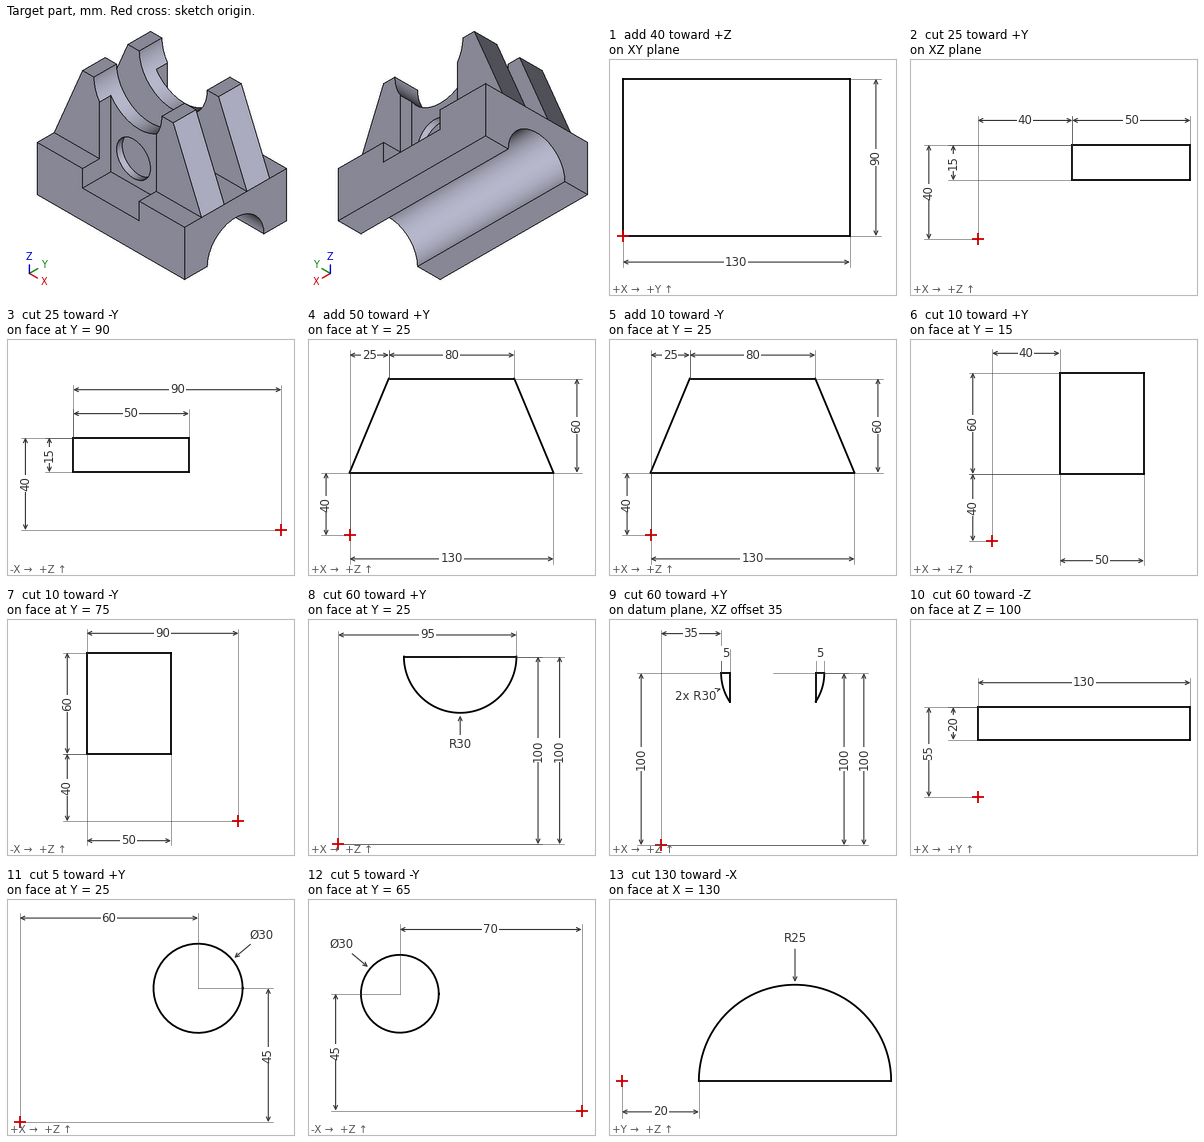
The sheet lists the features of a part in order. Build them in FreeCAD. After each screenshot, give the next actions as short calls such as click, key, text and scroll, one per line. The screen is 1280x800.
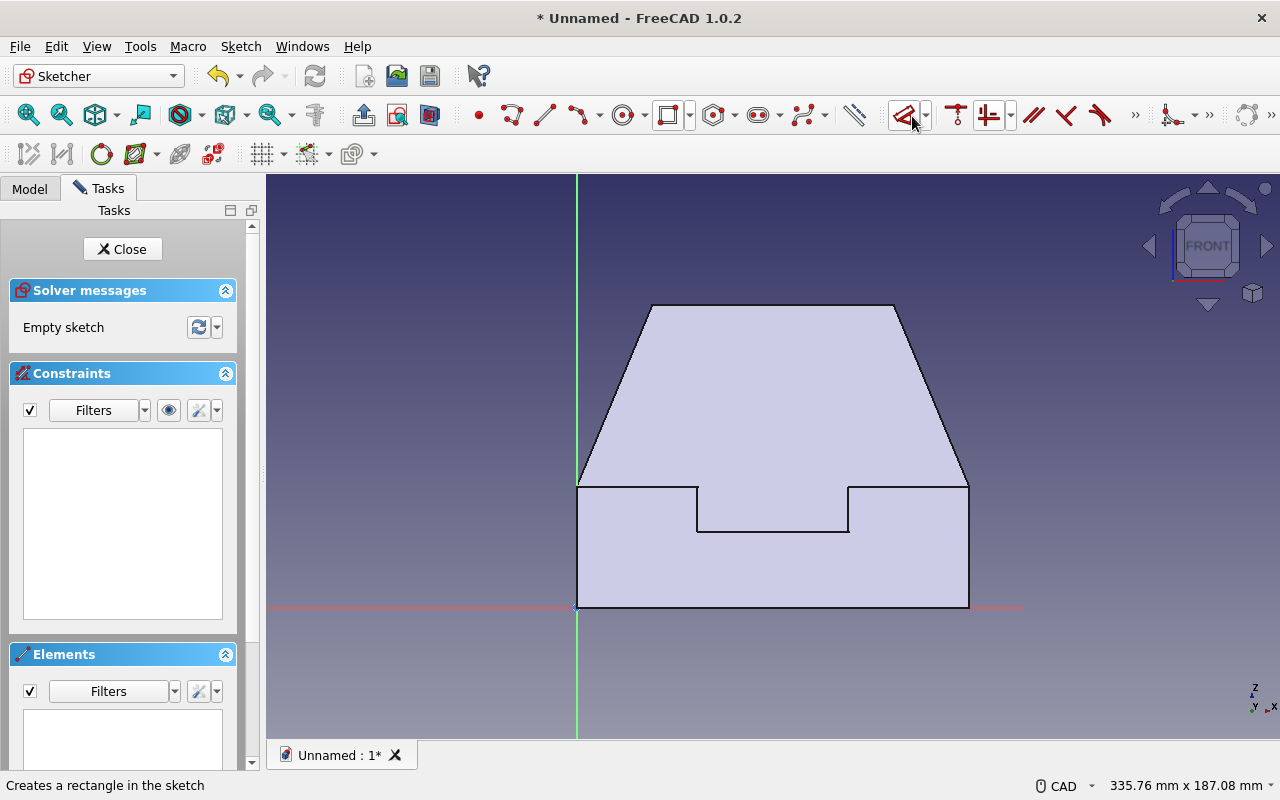
click(512, 116)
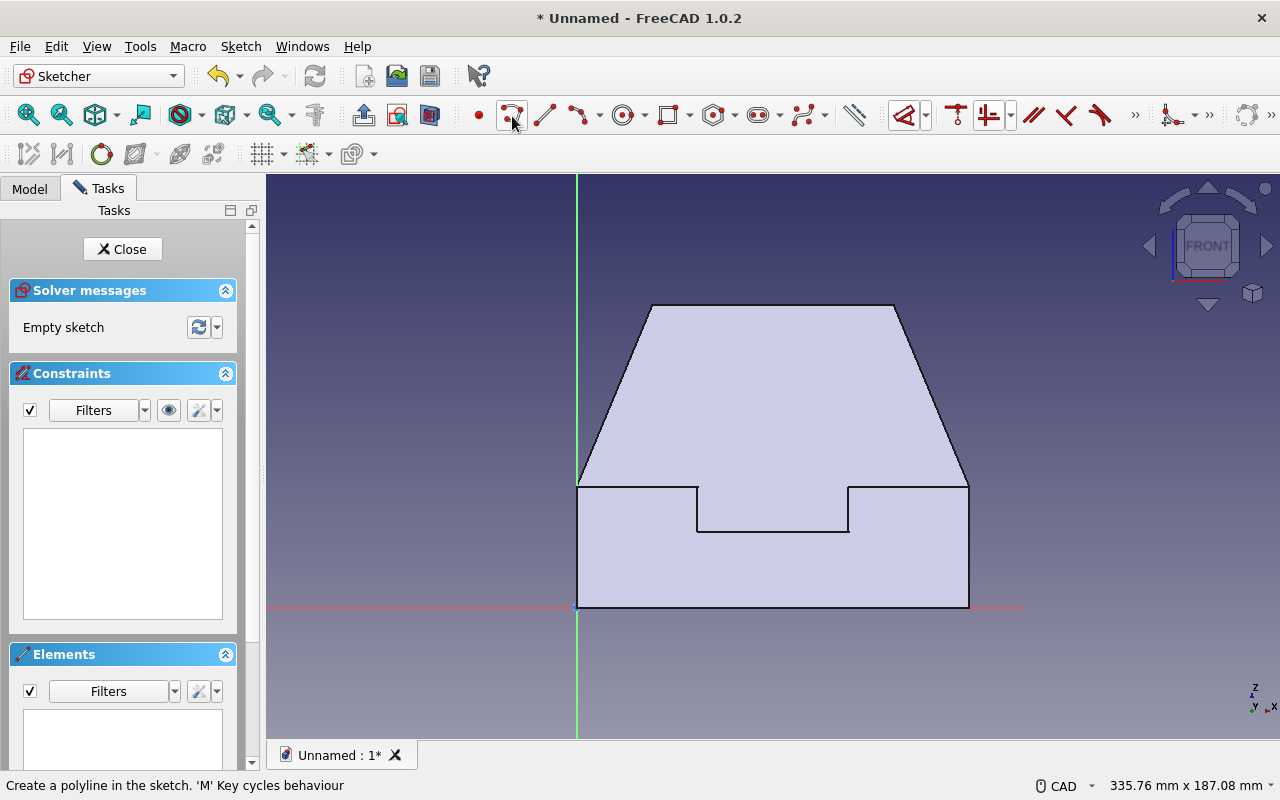
click(577, 487)
click(969, 487)
click(894, 305)
click(652, 305)
click(577, 488)
key(Escape)
key(Escape)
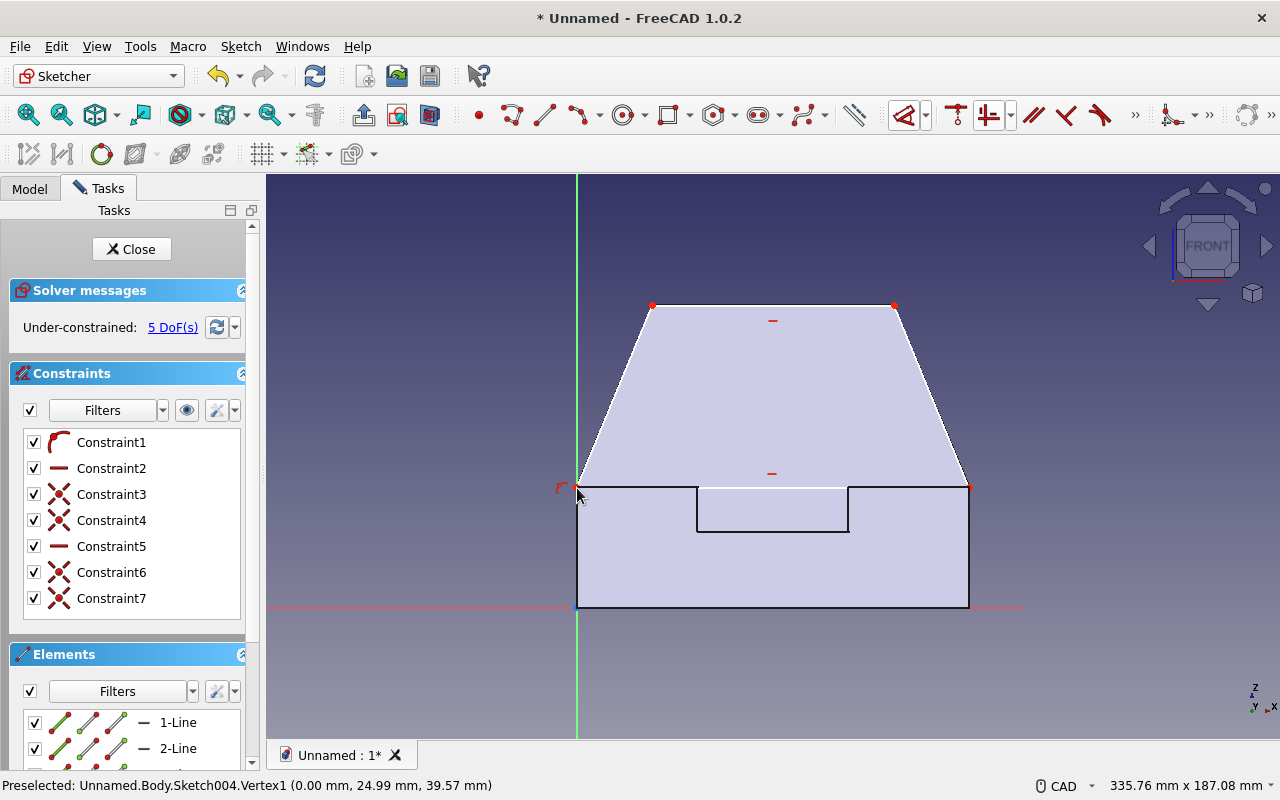
click(904, 116)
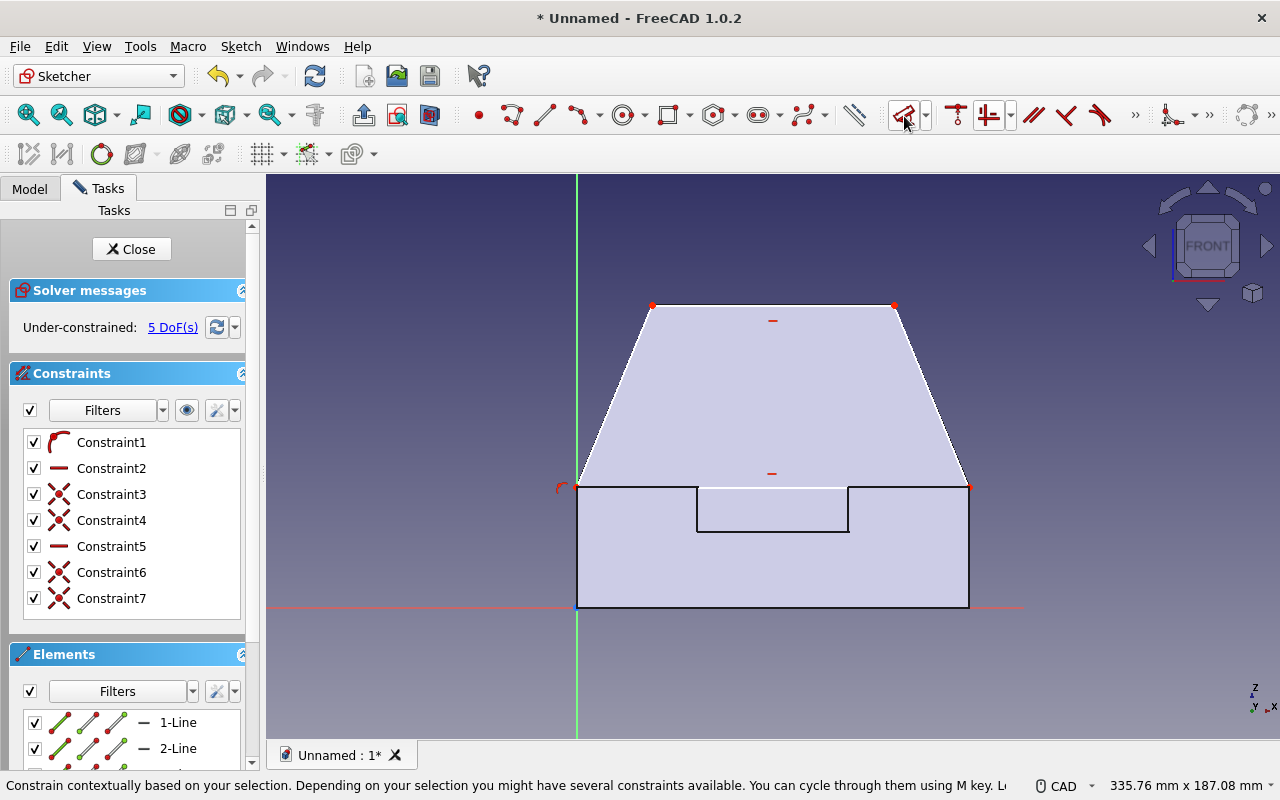
click(821, 306)
click(773, 272)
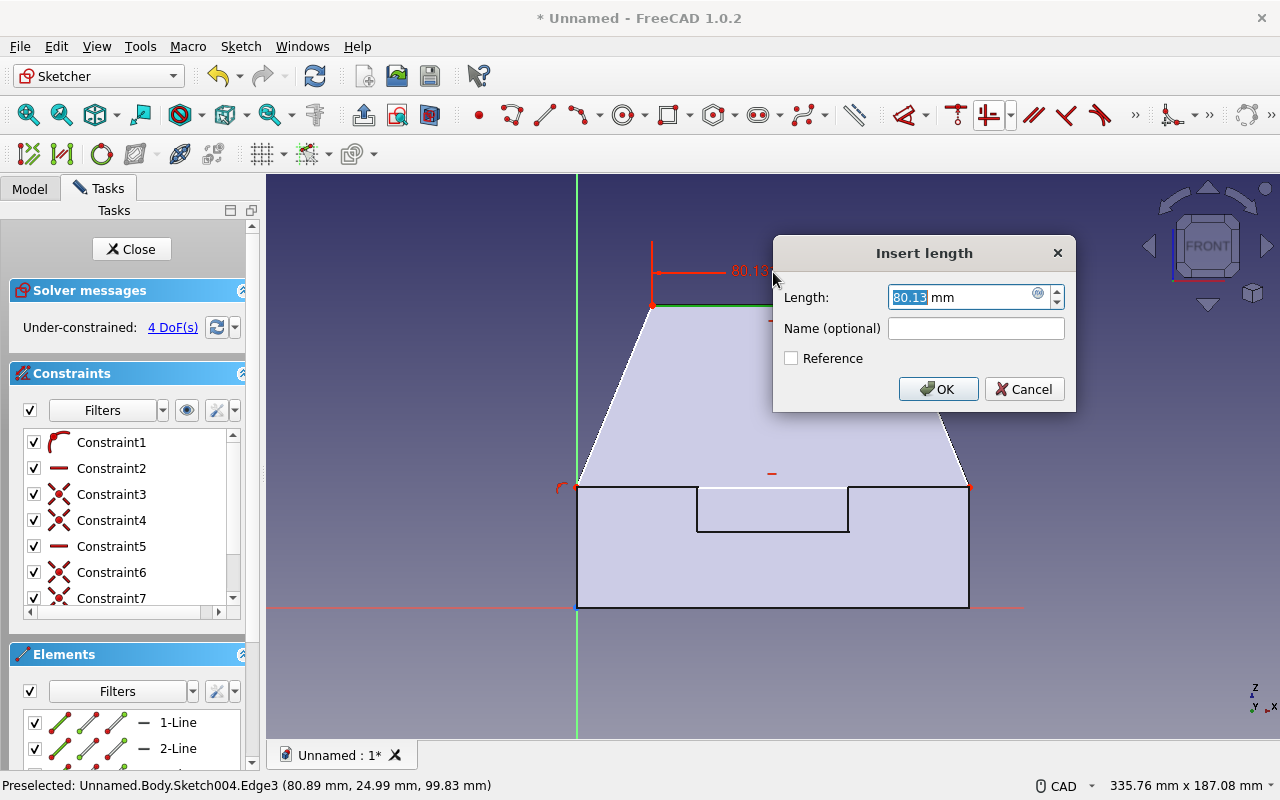
text(80)
key(Return)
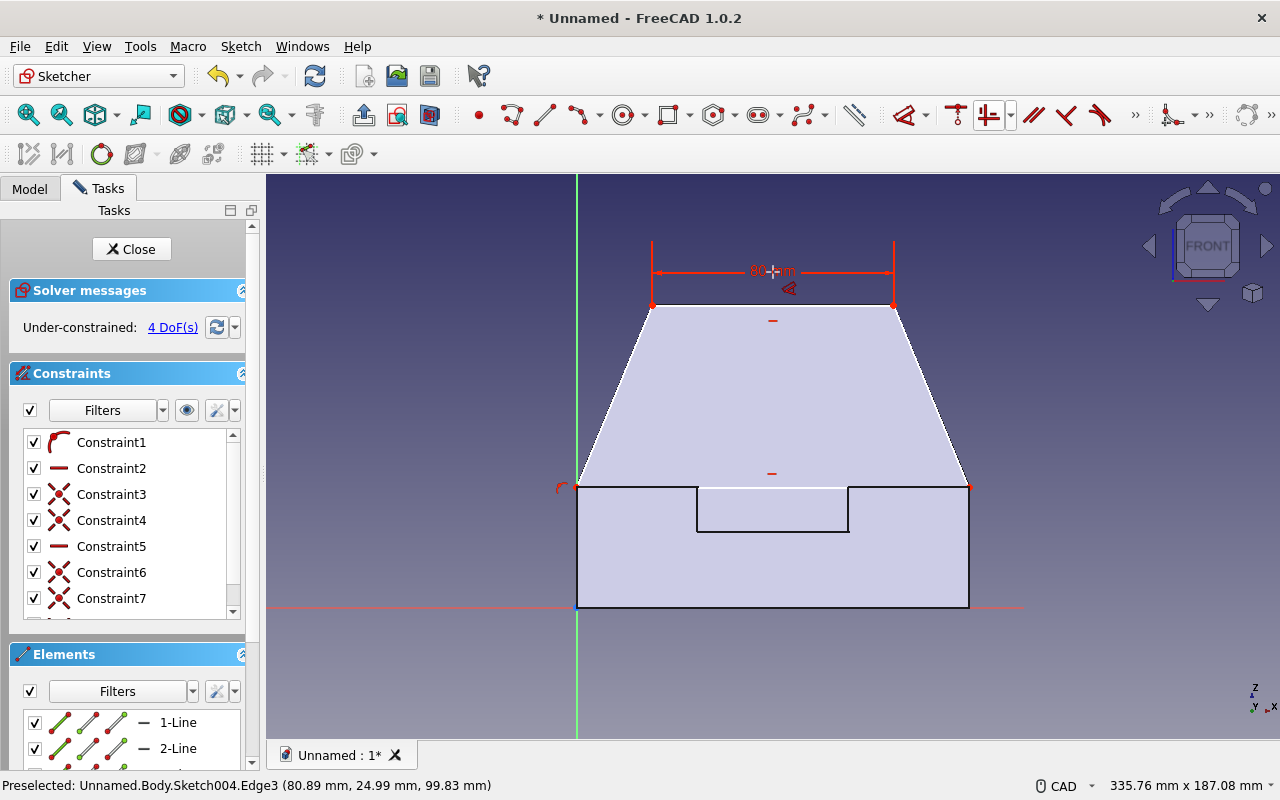
click(694, 488)
click(773, 522)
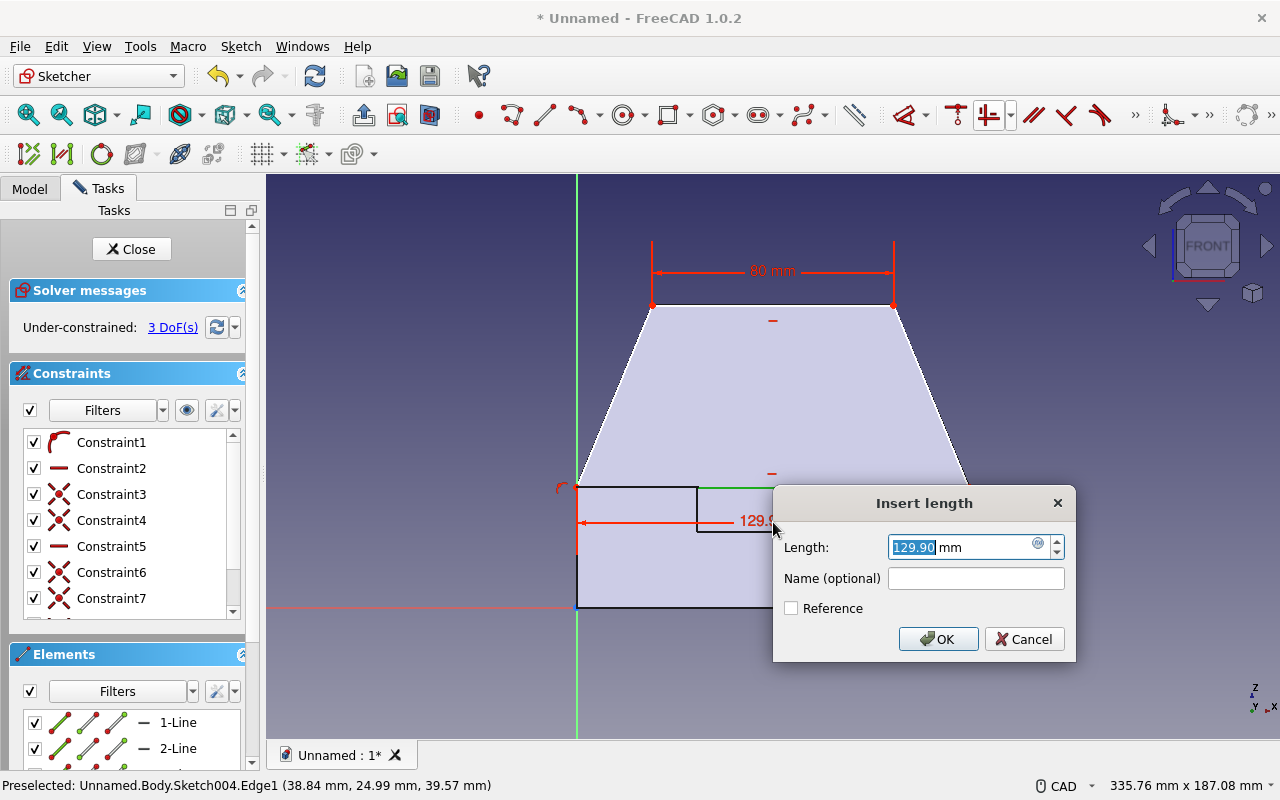
text(130)
key(Return)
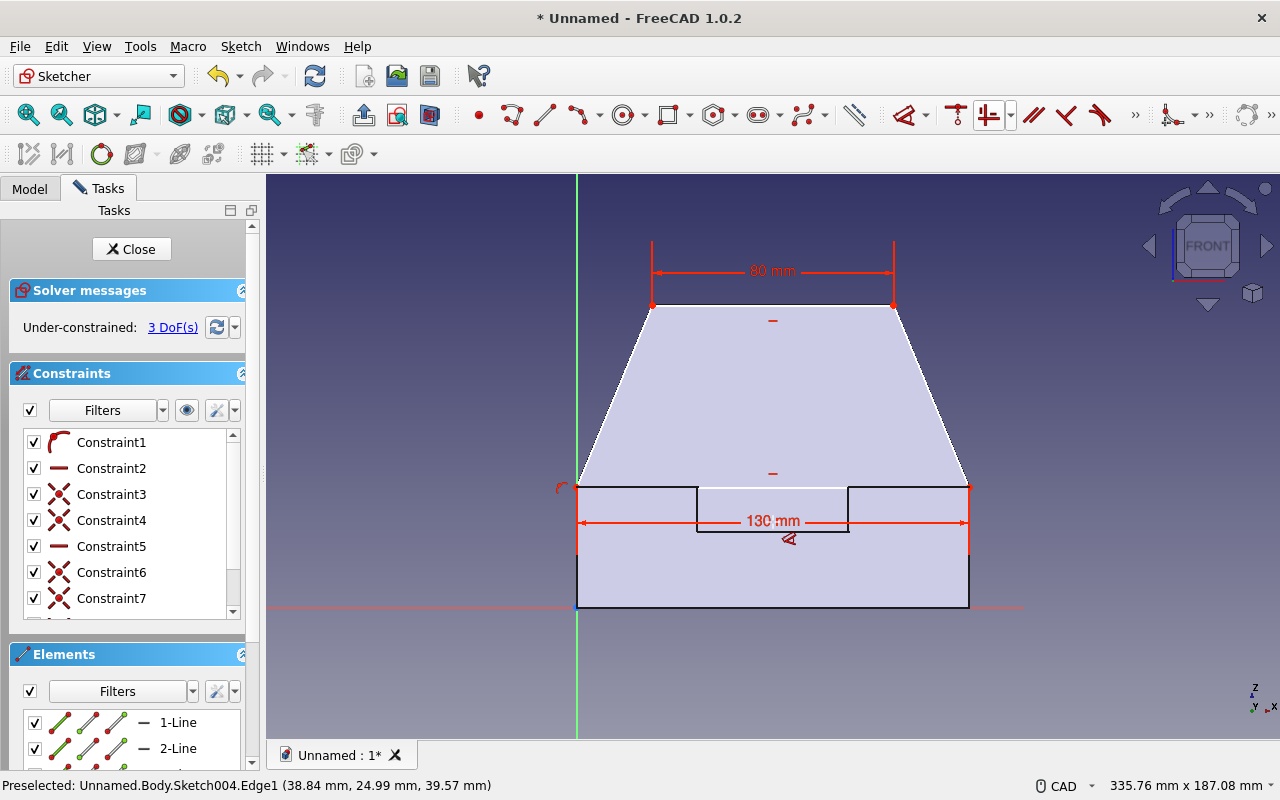
click(577, 488)
click(543, 548)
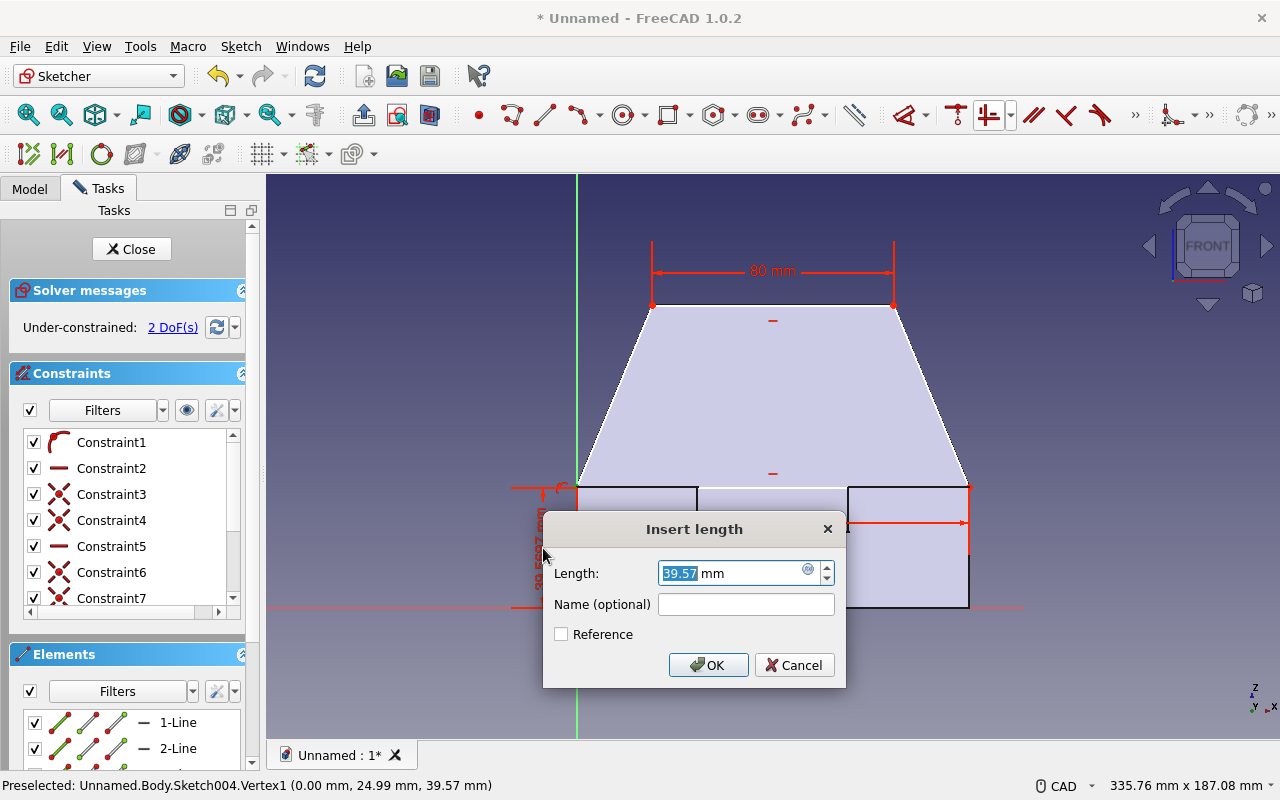
text(40)
key(Return)